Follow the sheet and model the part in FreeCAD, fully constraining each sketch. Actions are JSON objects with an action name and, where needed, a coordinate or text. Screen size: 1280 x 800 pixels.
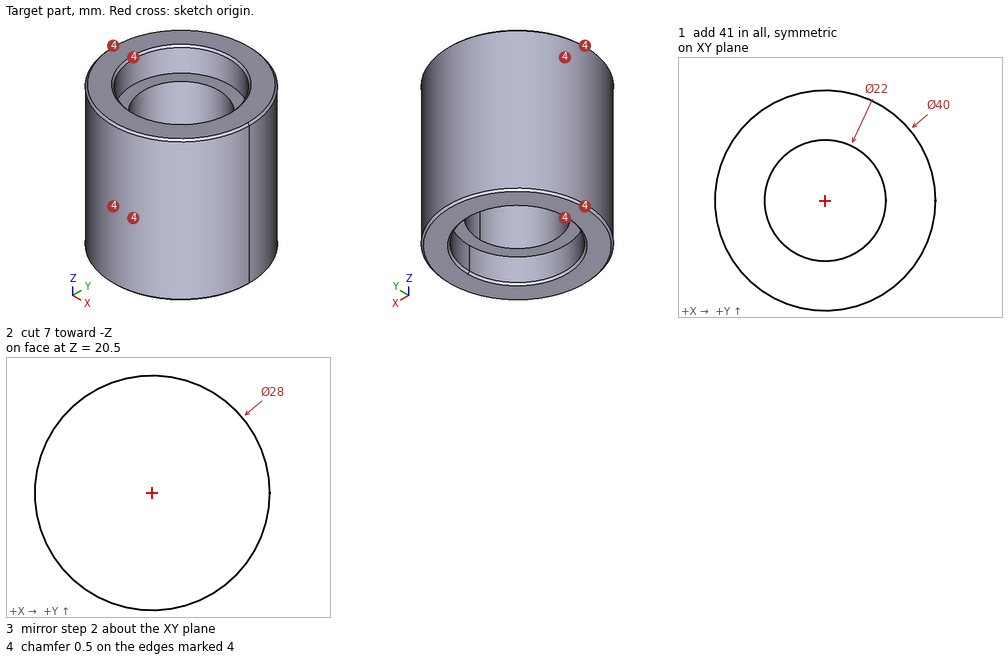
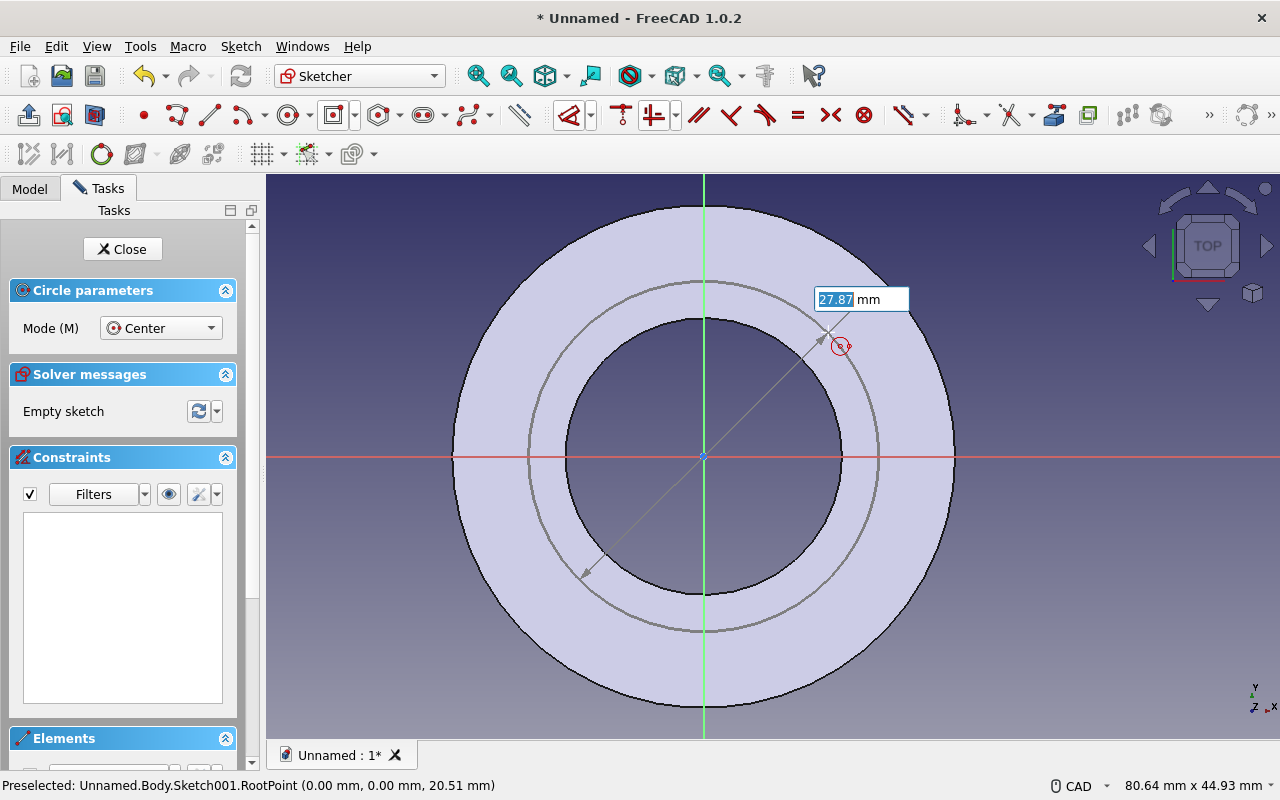
{"action": "type", "text": "28"}
{"action": "key", "text": "Return"}
{"action": "key", "text": "Escape"}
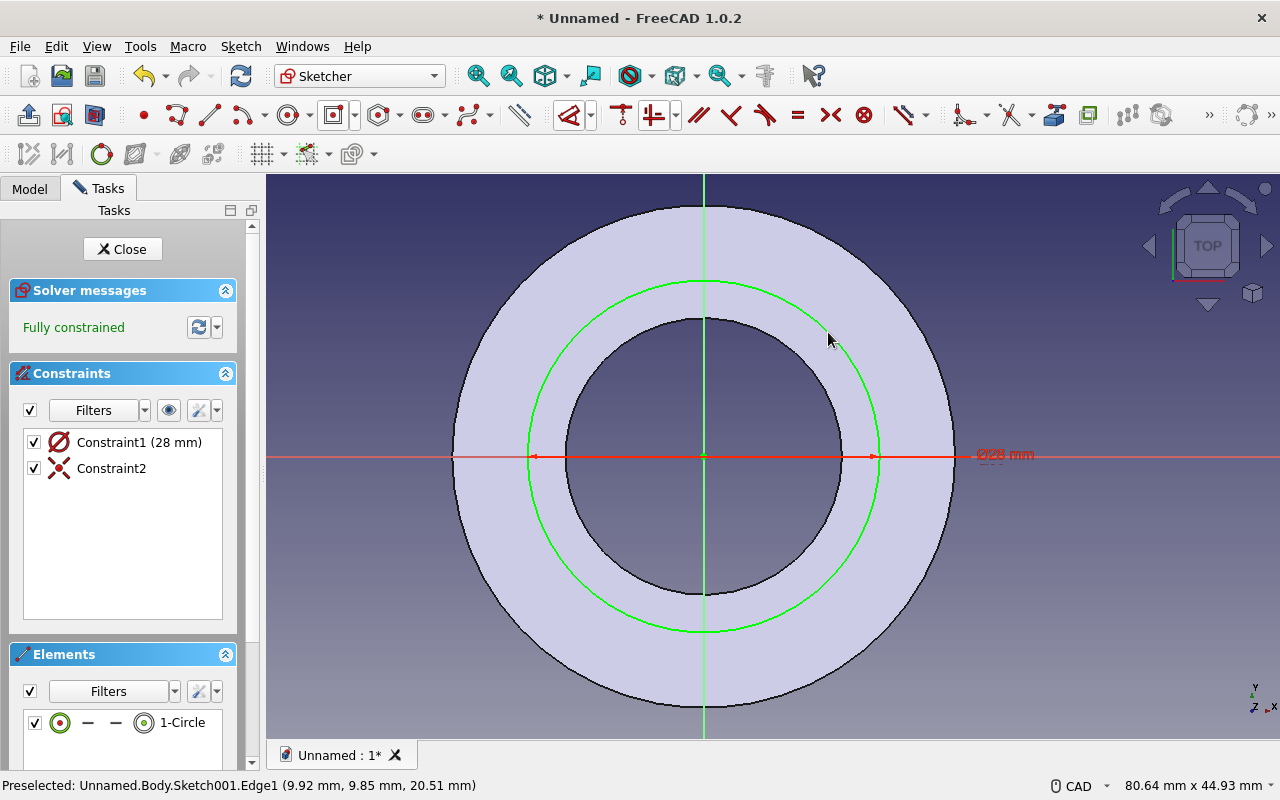
{"action": "left_click", "coordinate": [123, 249]}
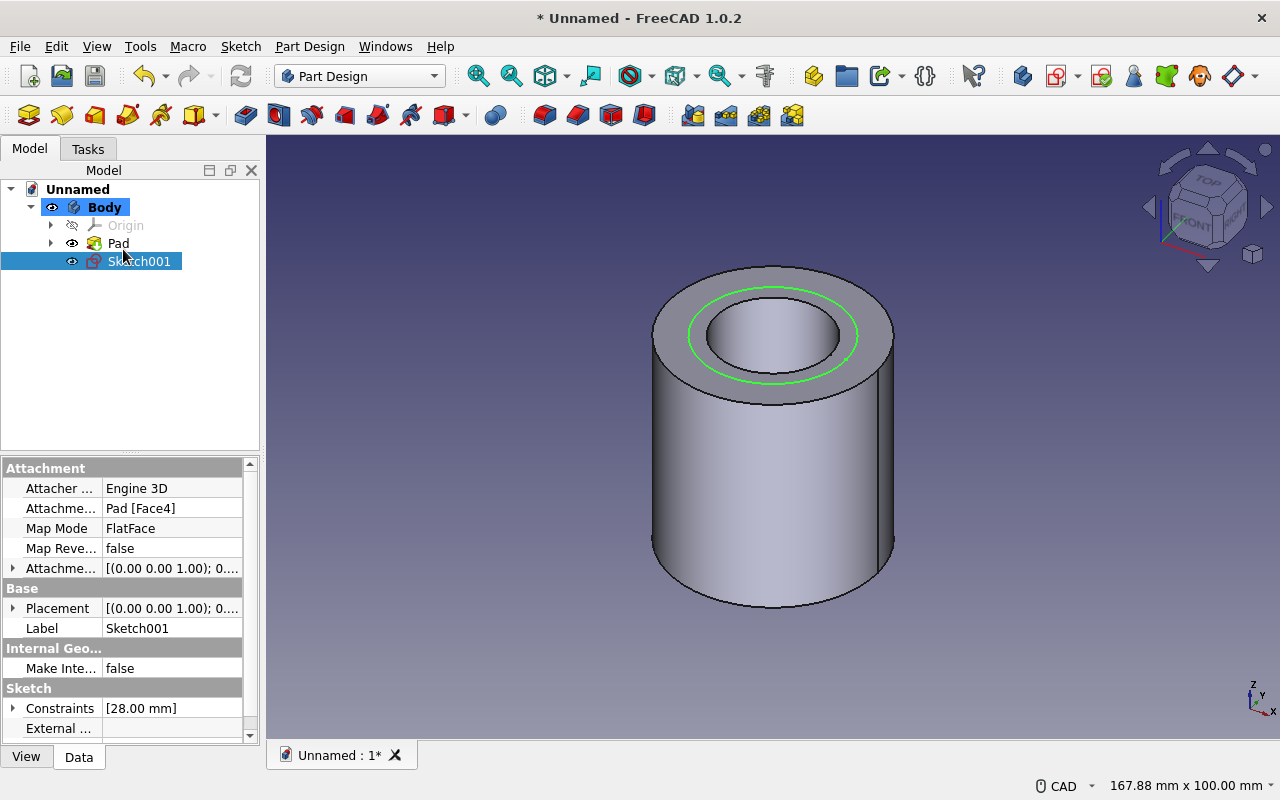
{"action": "left_click", "coordinate": [246, 116]}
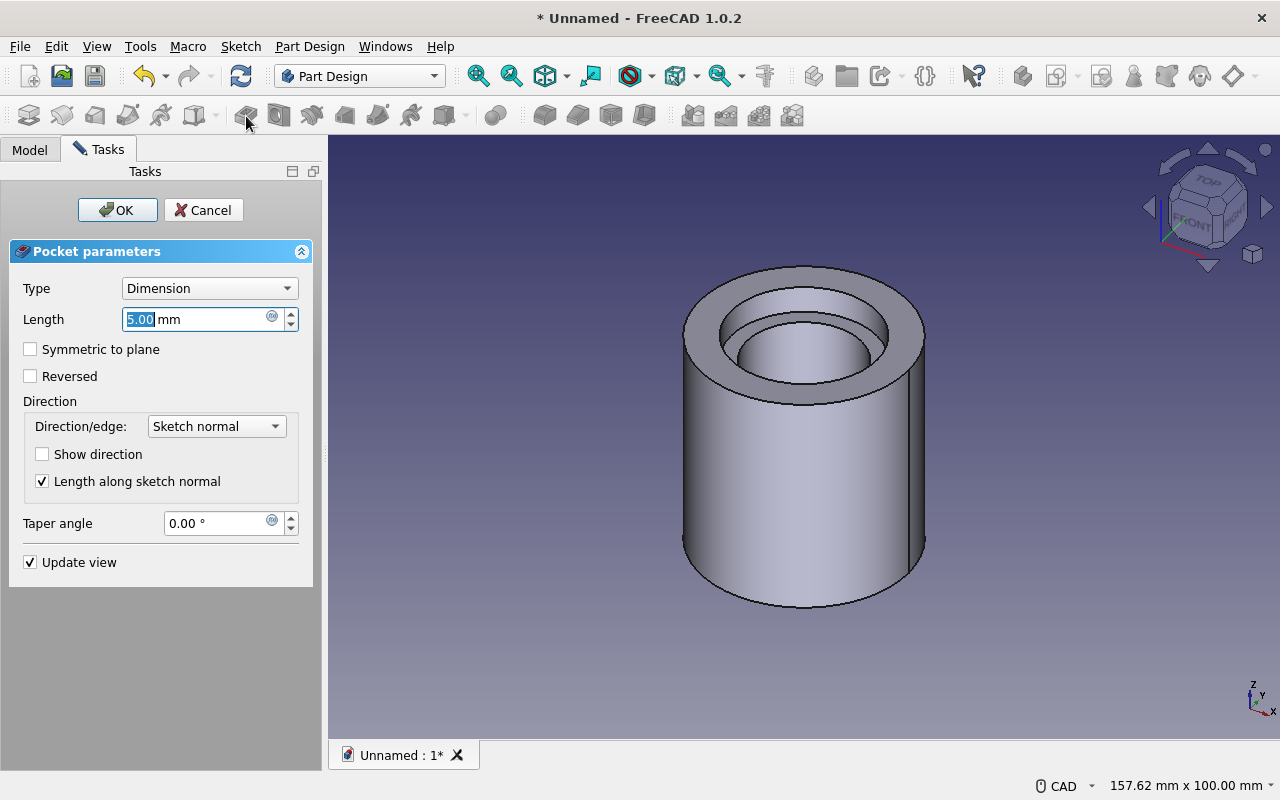
{"action": "type", "text": "7"}
{"action": "key", "text": "Tab"}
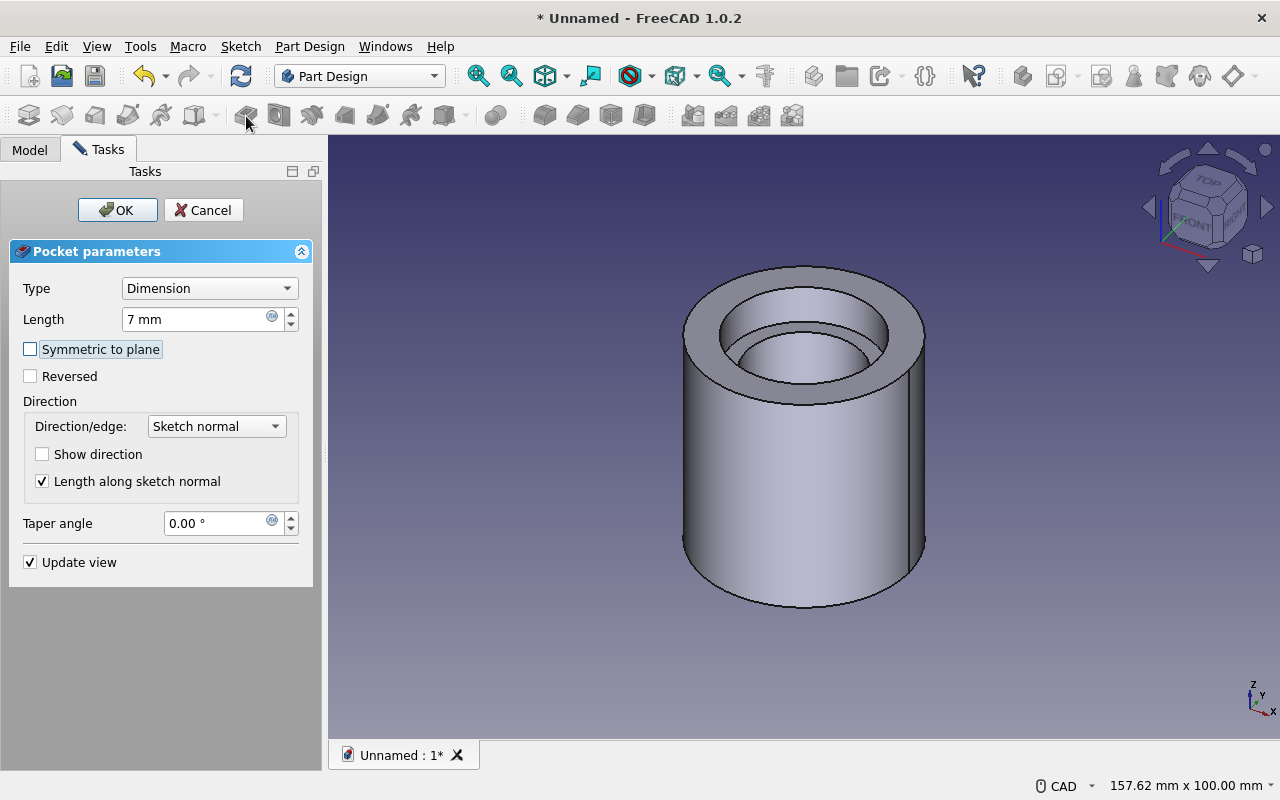
{"action": "left_click", "coordinate": [118, 210]}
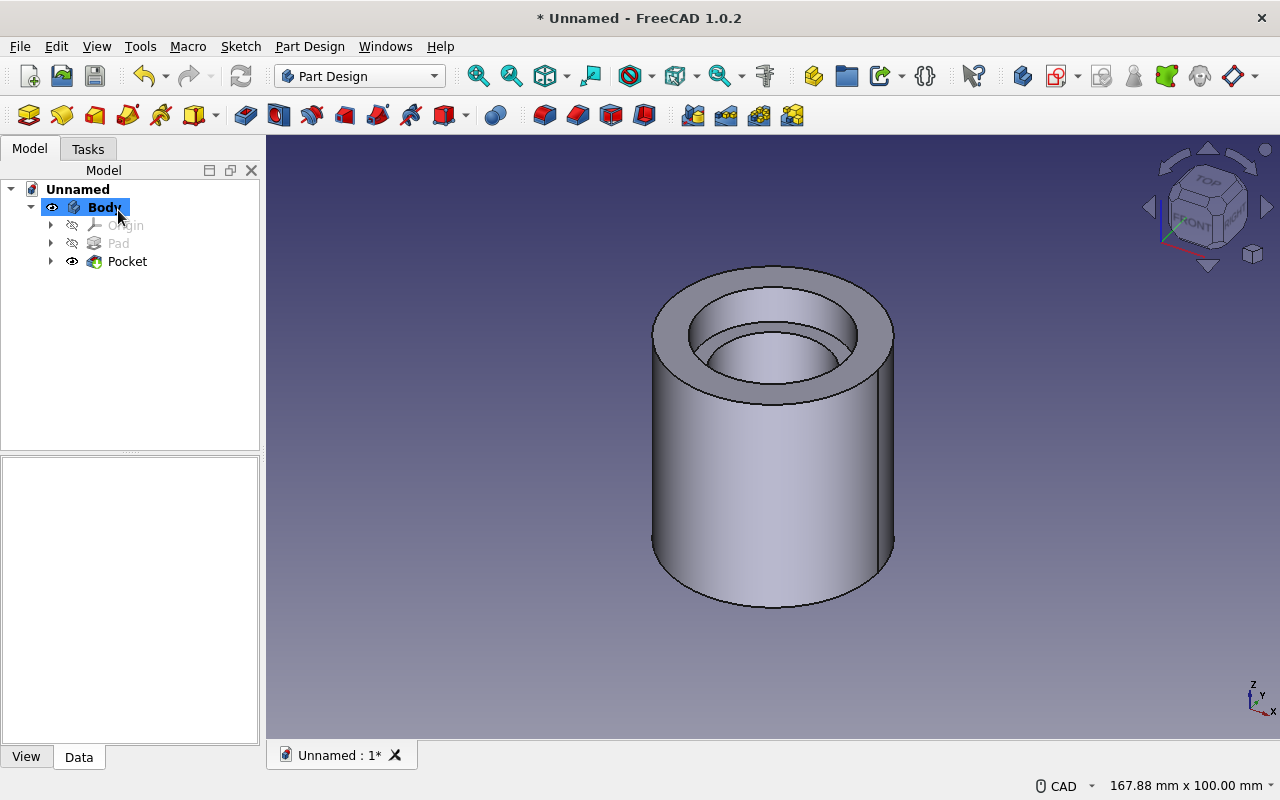
{"action": "left_click", "coordinate": [117, 261]}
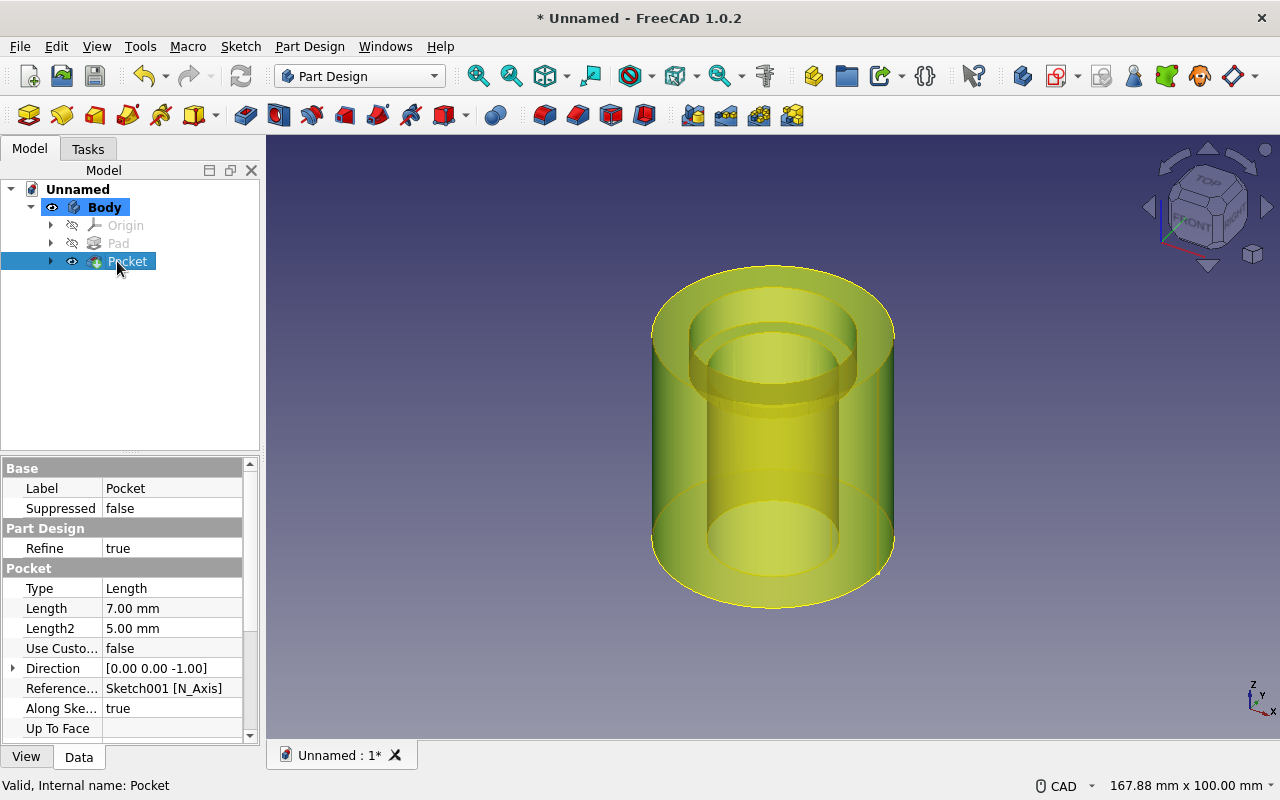
{"action": "left_click", "coordinate": [693, 116]}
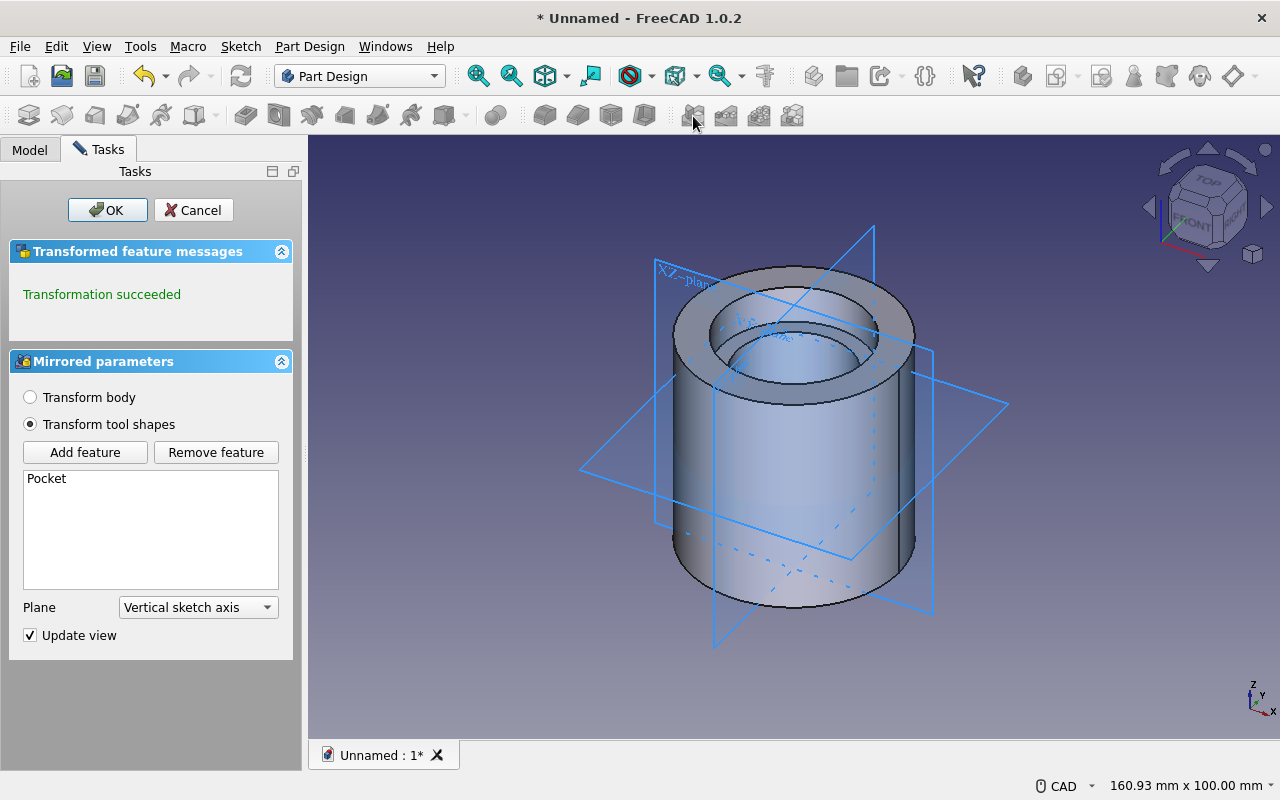
{"action": "left_click", "coordinate": [199, 608]}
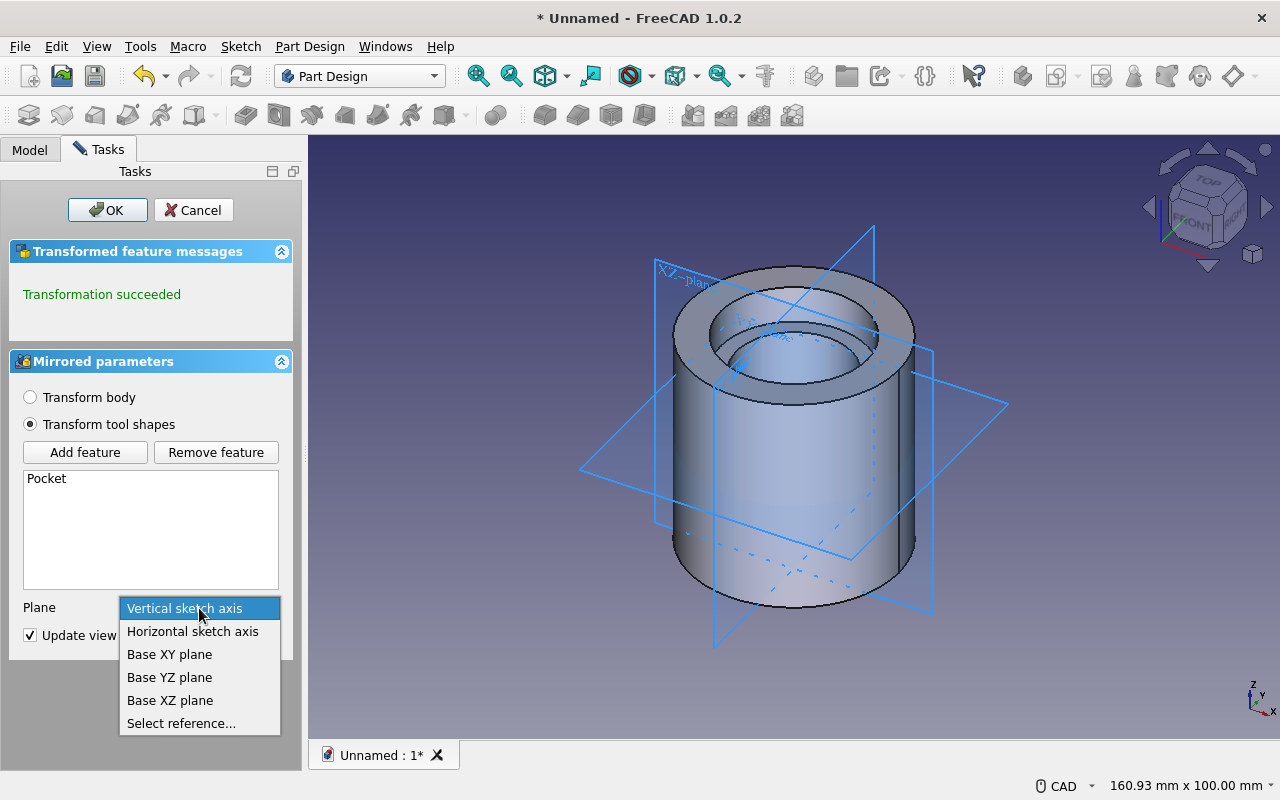
{"action": "left_click", "coordinate": [198, 654]}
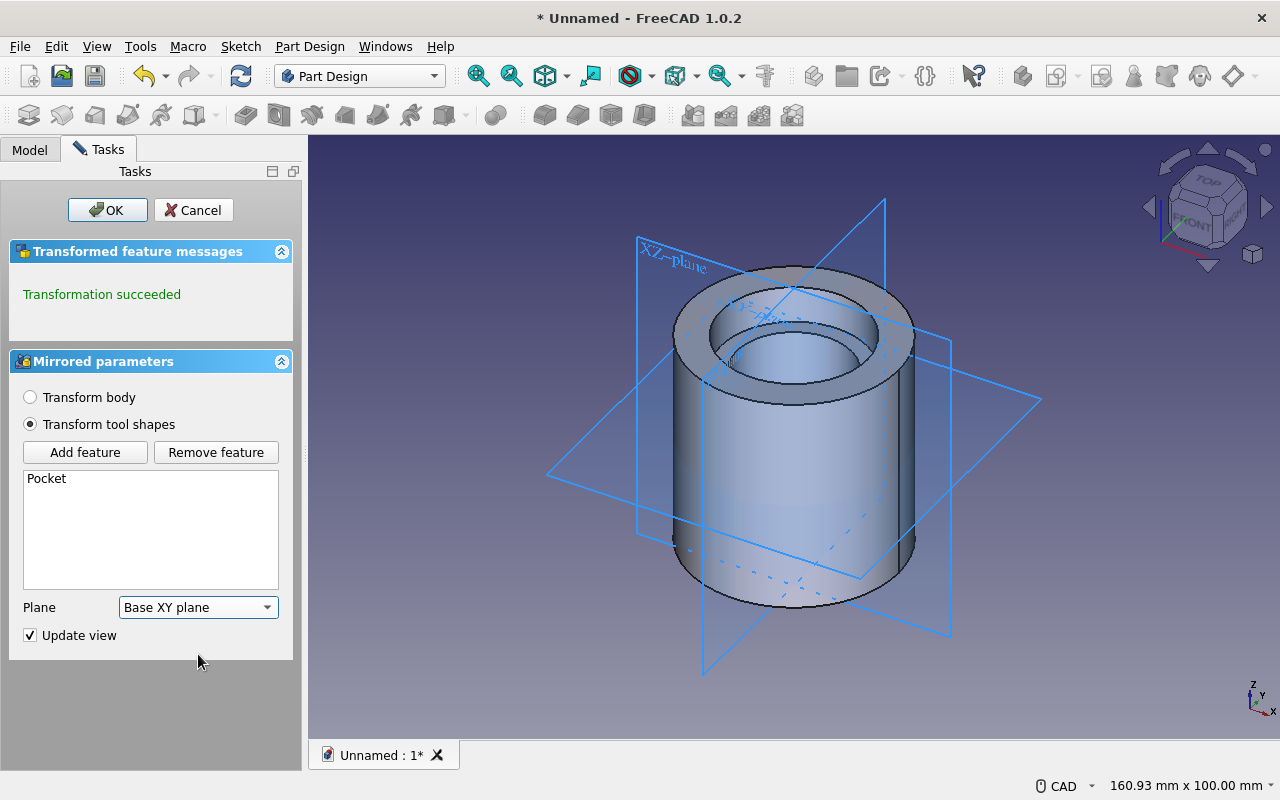
{"action": "left_click", "coordinate": [108, 210]}